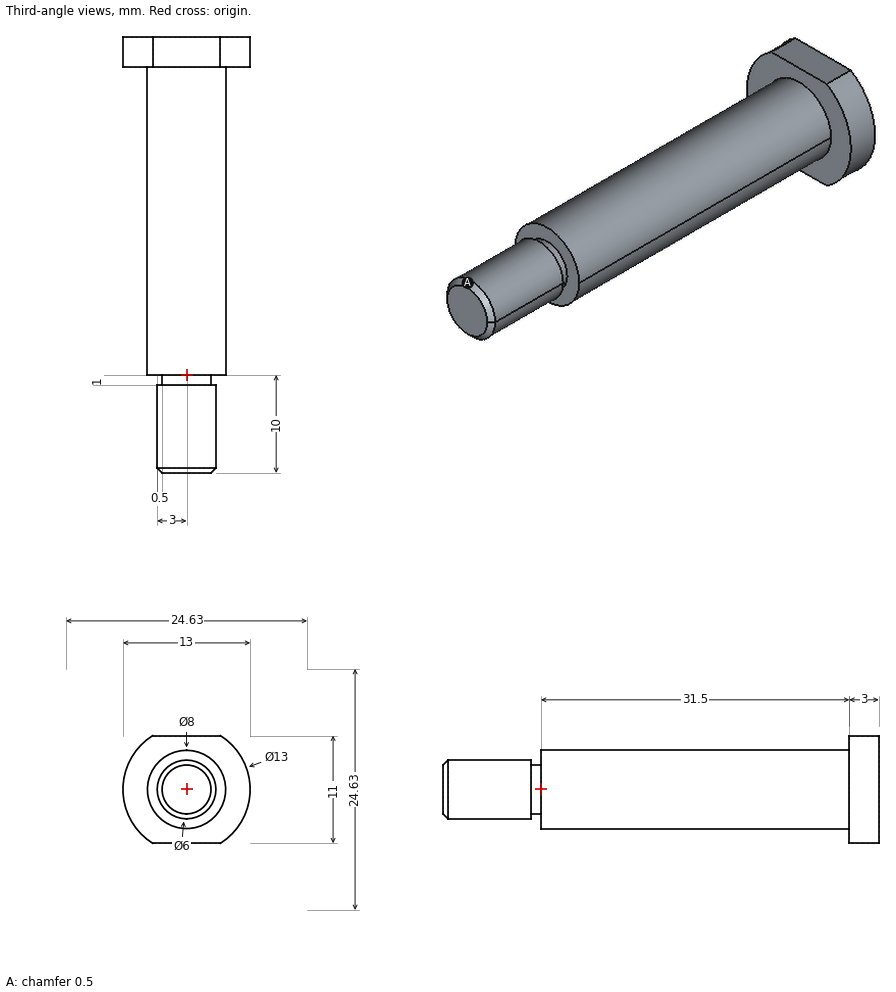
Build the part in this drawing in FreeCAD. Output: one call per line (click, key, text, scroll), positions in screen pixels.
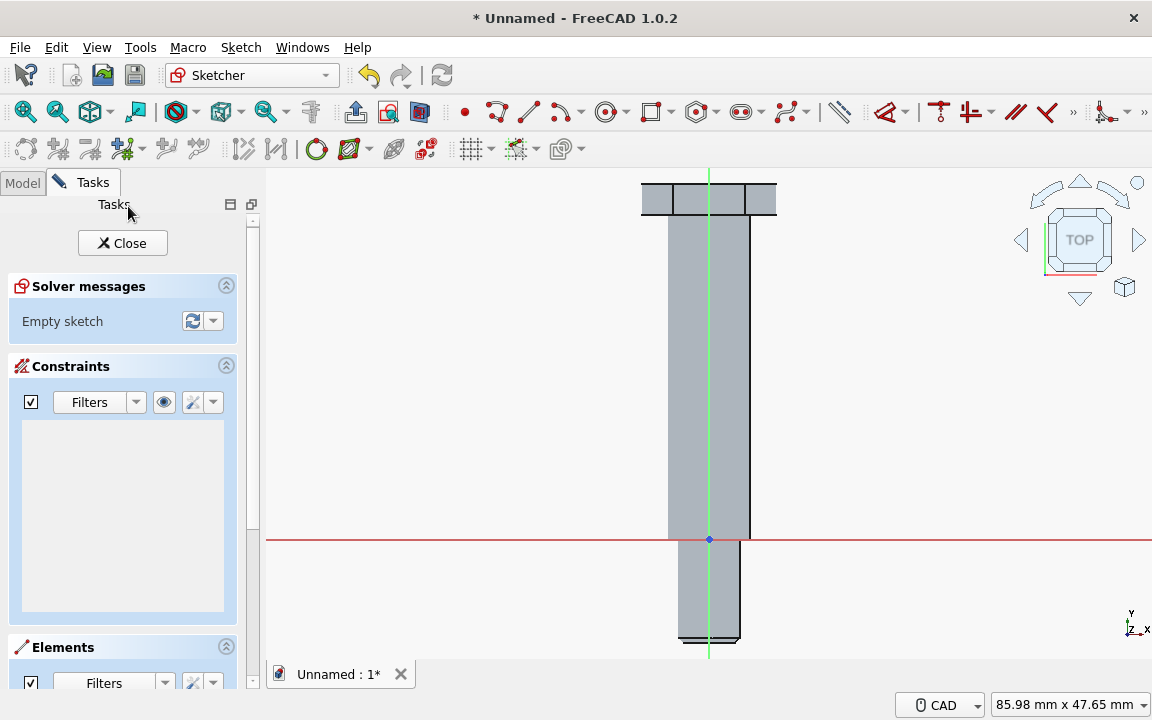
scroll(683, 552, up, 15)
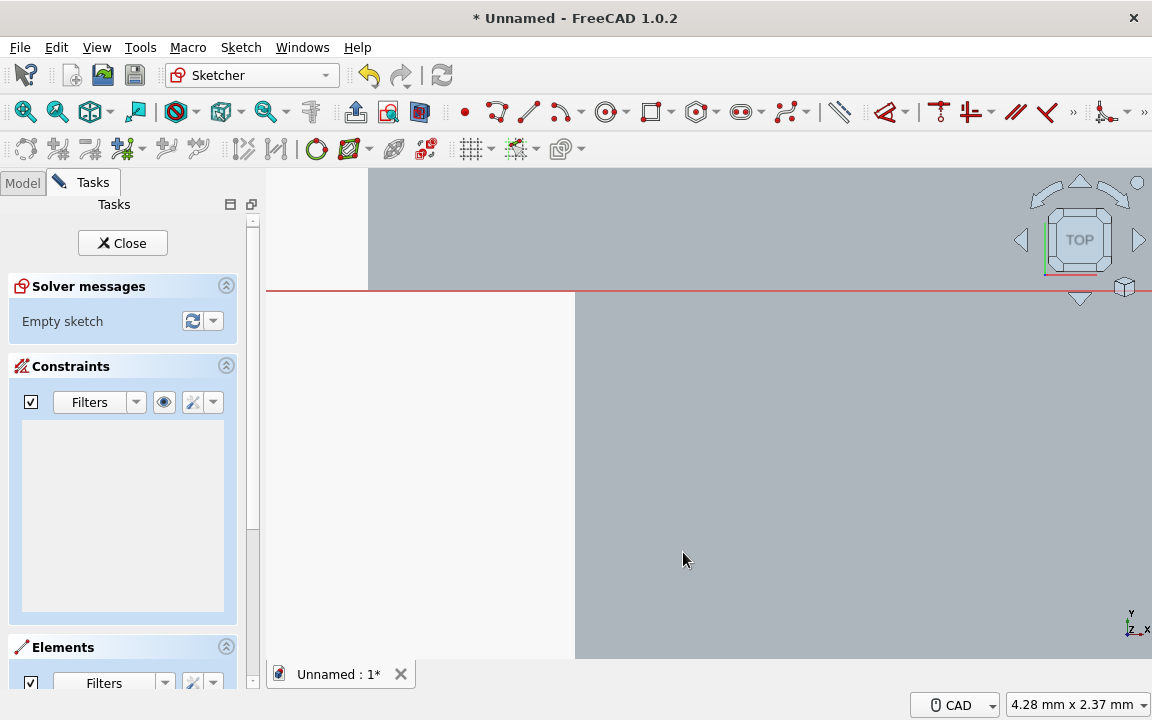
scroll(600, 355, up, 2)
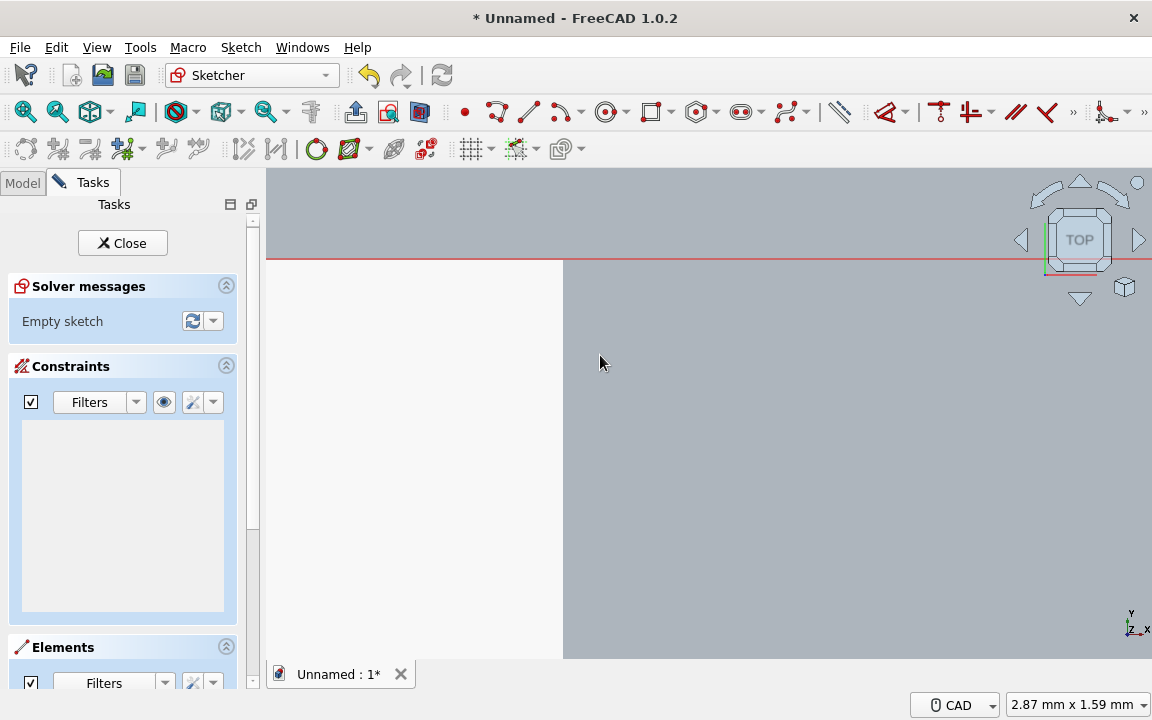
key(g)
key(r)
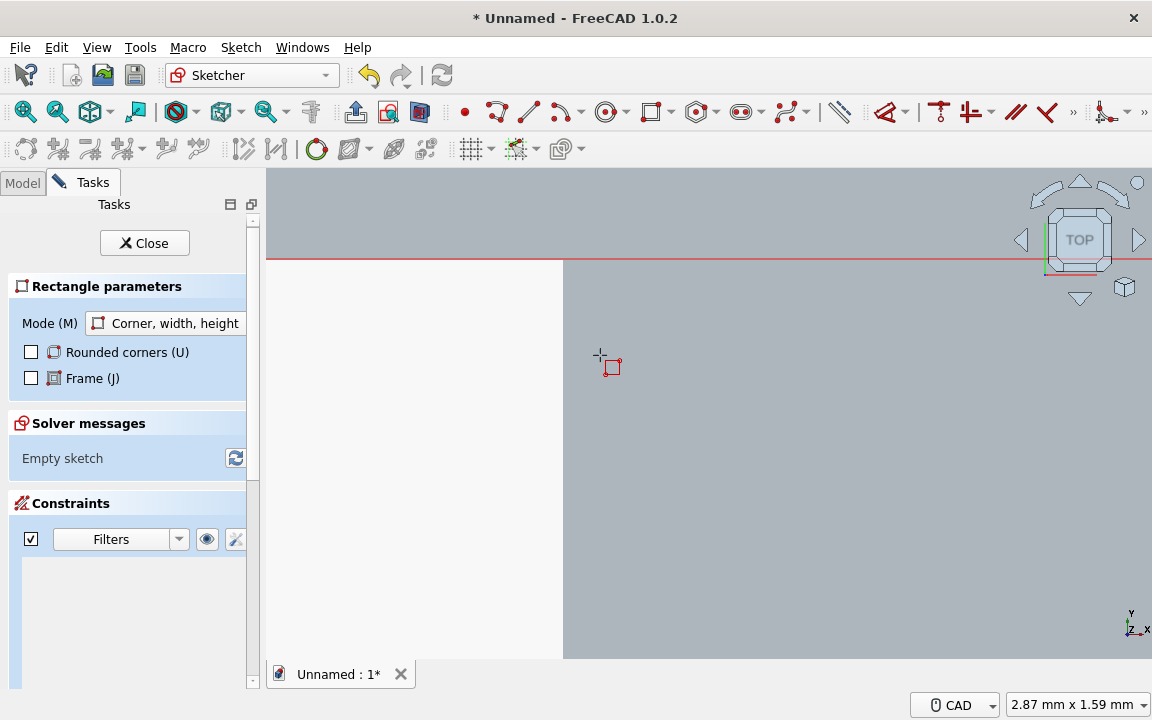
click(563, 259)
move(717, 568)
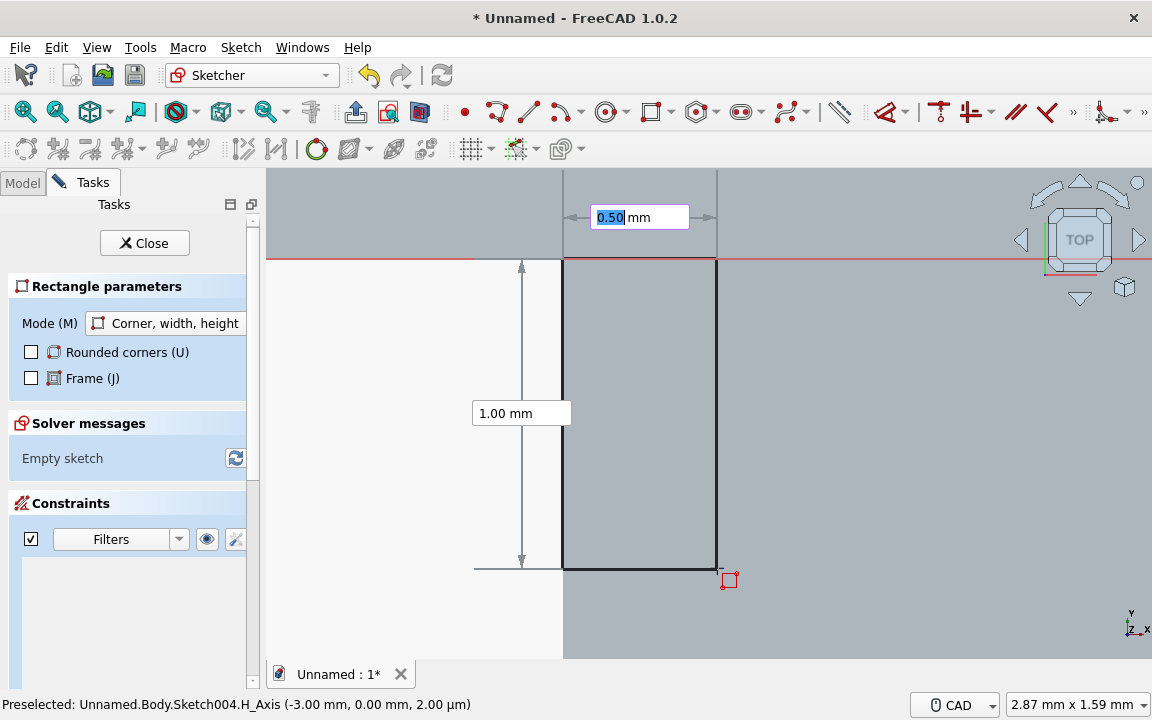
text(0.5)
key(Tab)
text(1)
key(Return)
key(Escape)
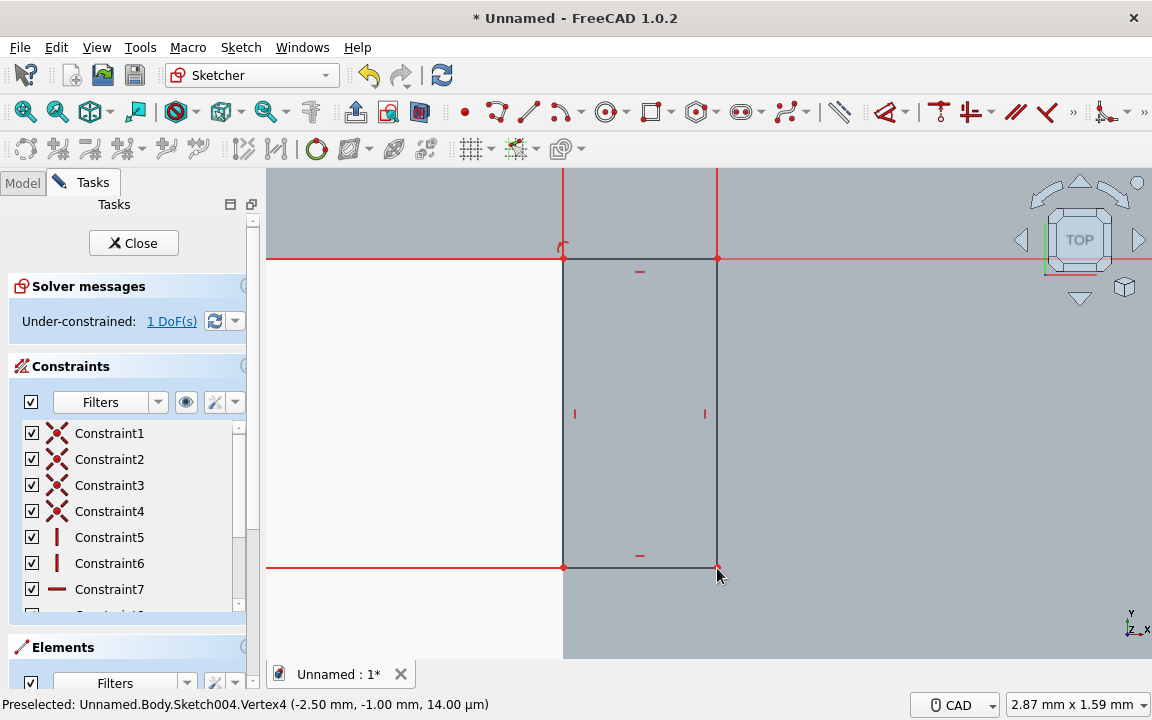
key(d)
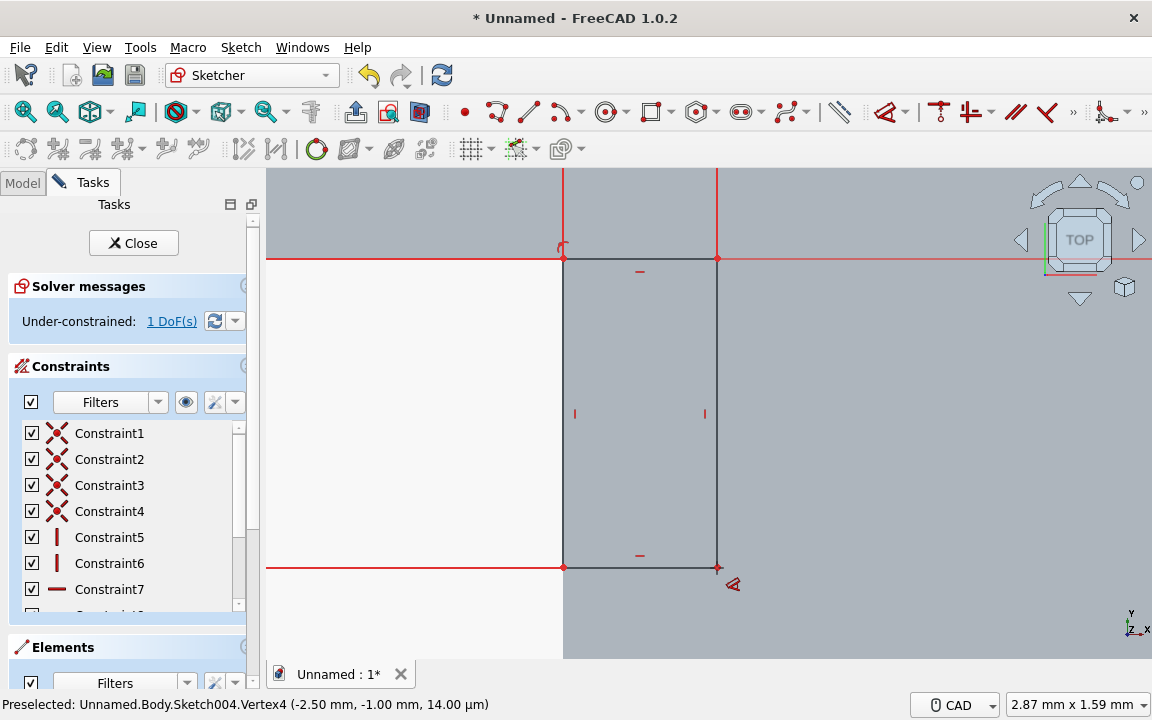
click(563, 259)
click(775, 225)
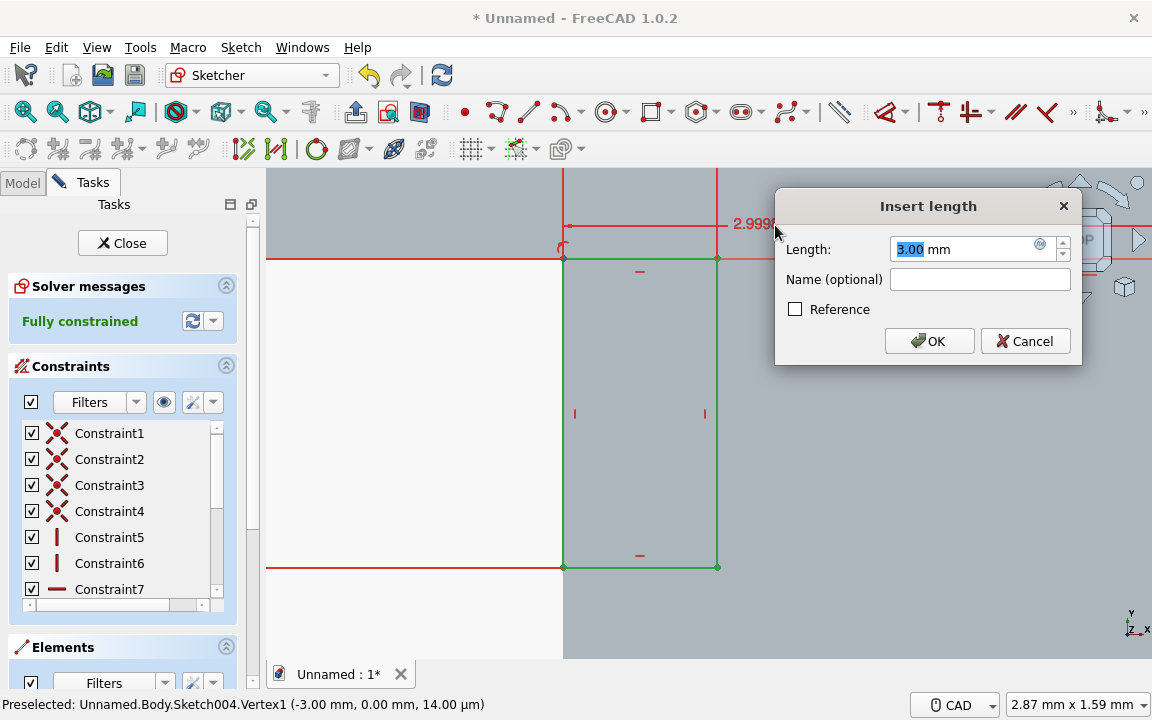
text(3)
key(Return)
key(Escape)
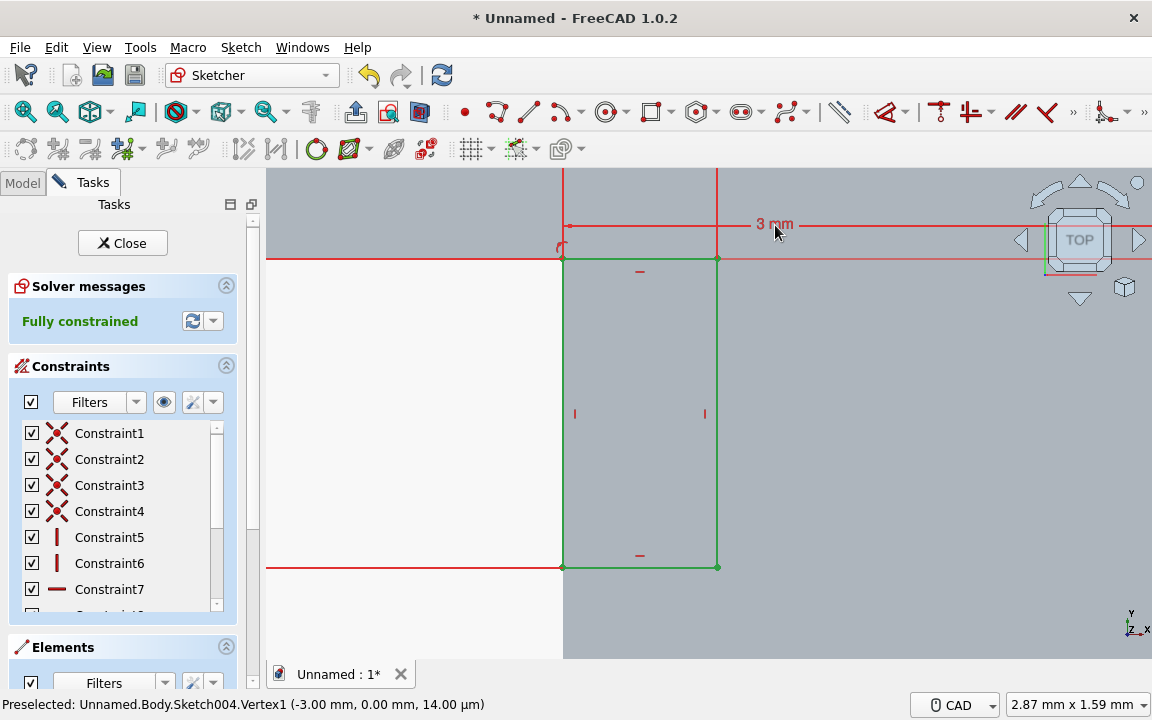
click(123, 243)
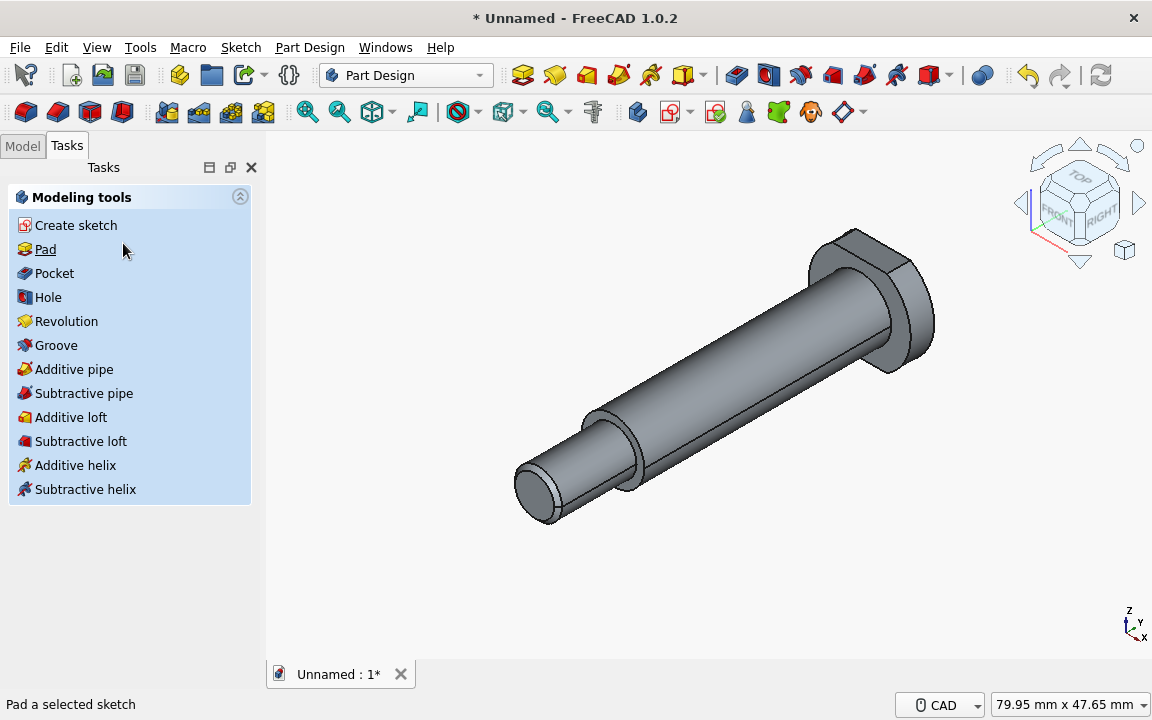
click(802, 76)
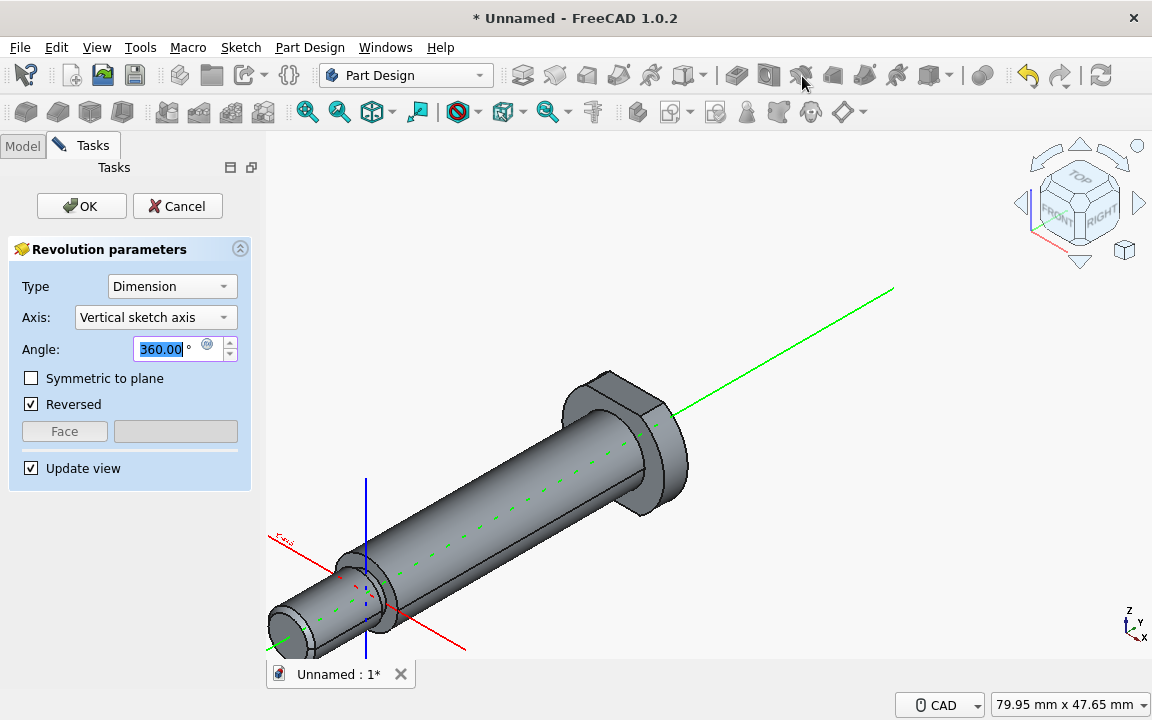
click(82, 206)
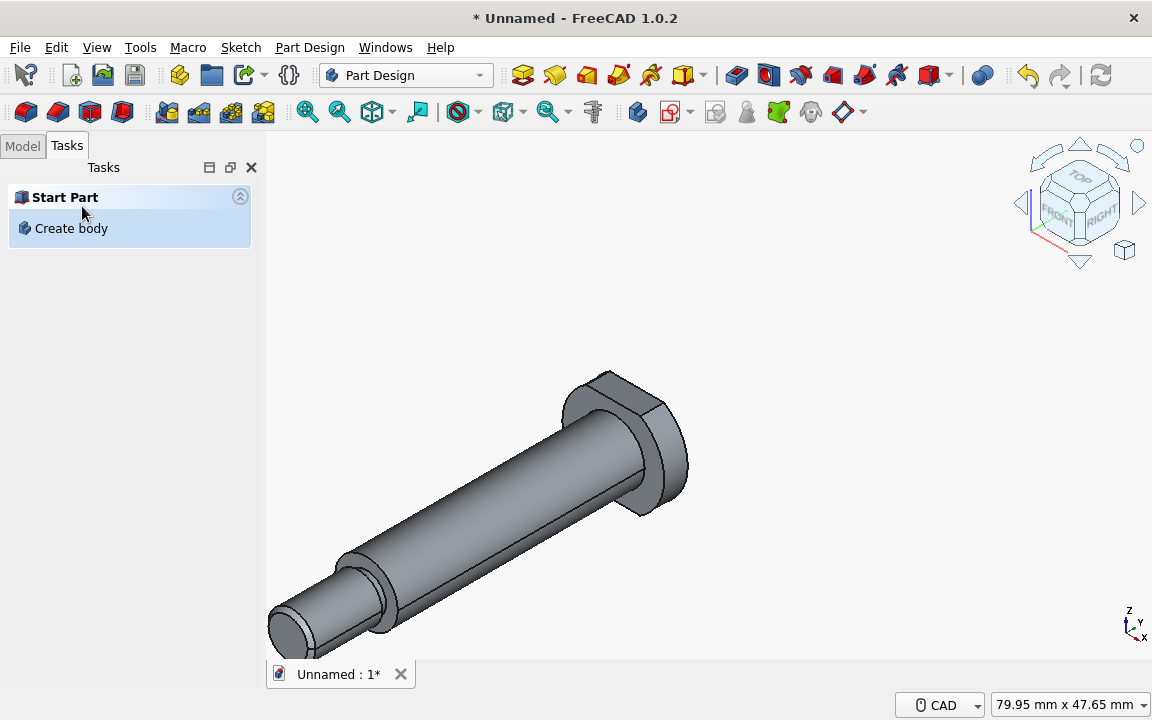
key(v)
key(f)